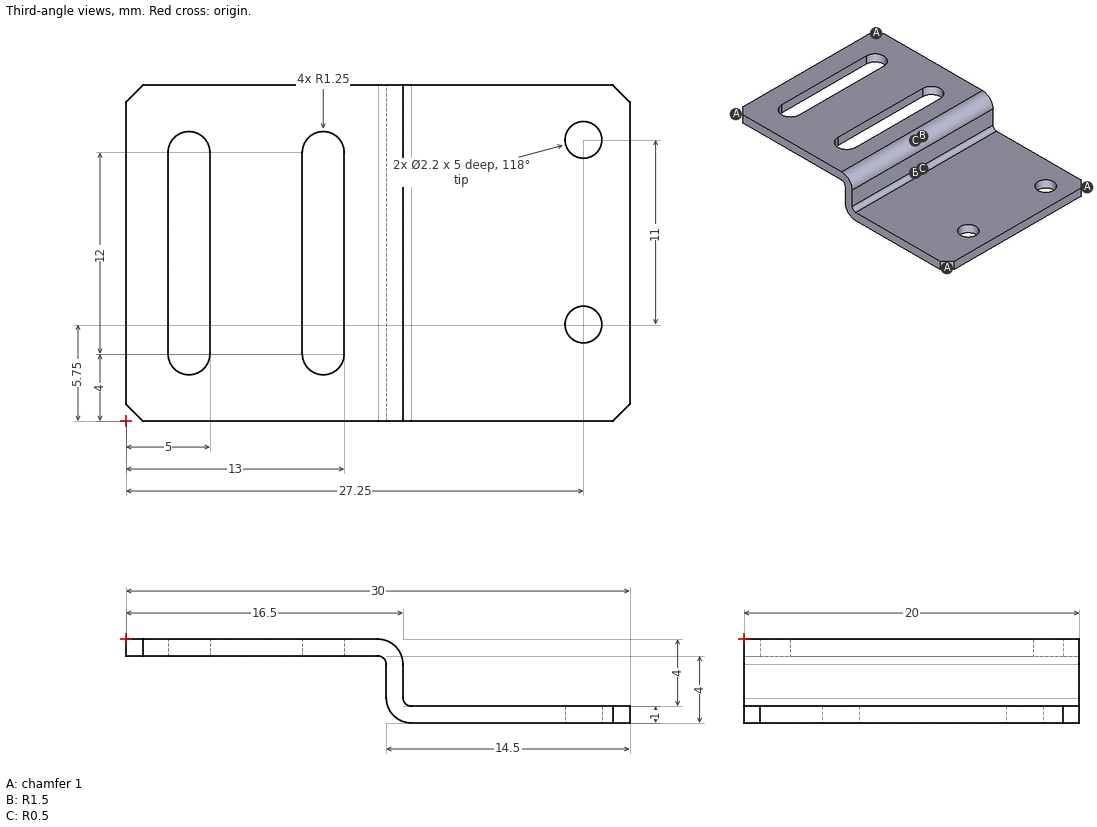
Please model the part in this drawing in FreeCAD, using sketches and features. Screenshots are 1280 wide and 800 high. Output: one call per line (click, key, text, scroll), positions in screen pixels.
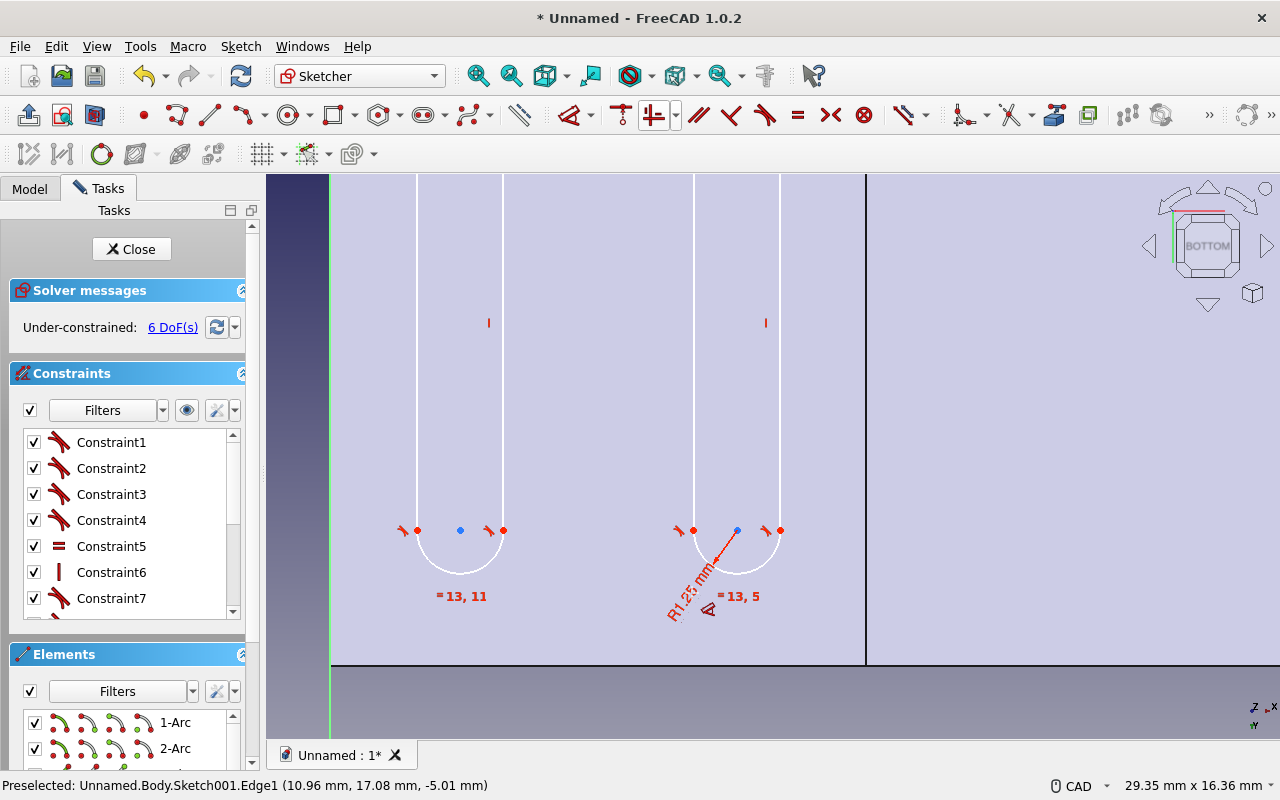
click(694, 406)
click(728, 366)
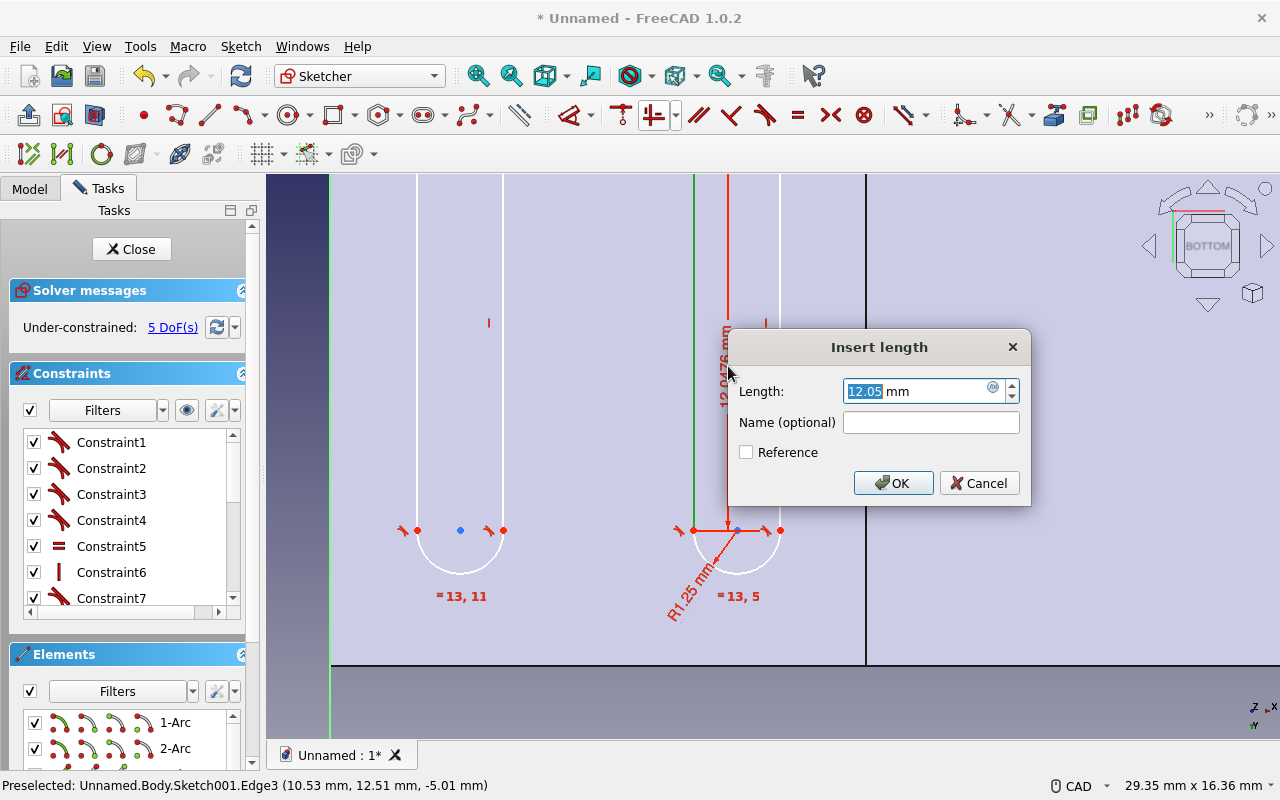
text(12)
key(Return)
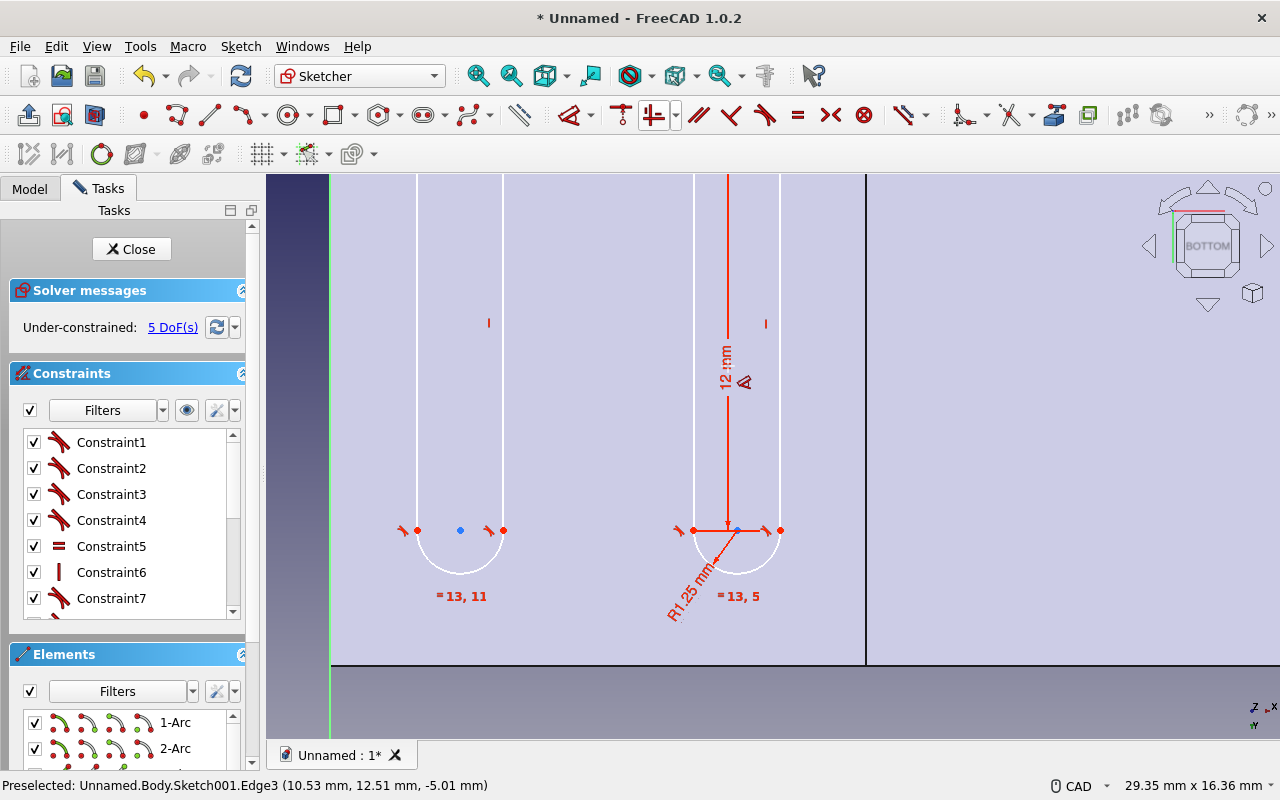
click(417, 406)
click(383, 366)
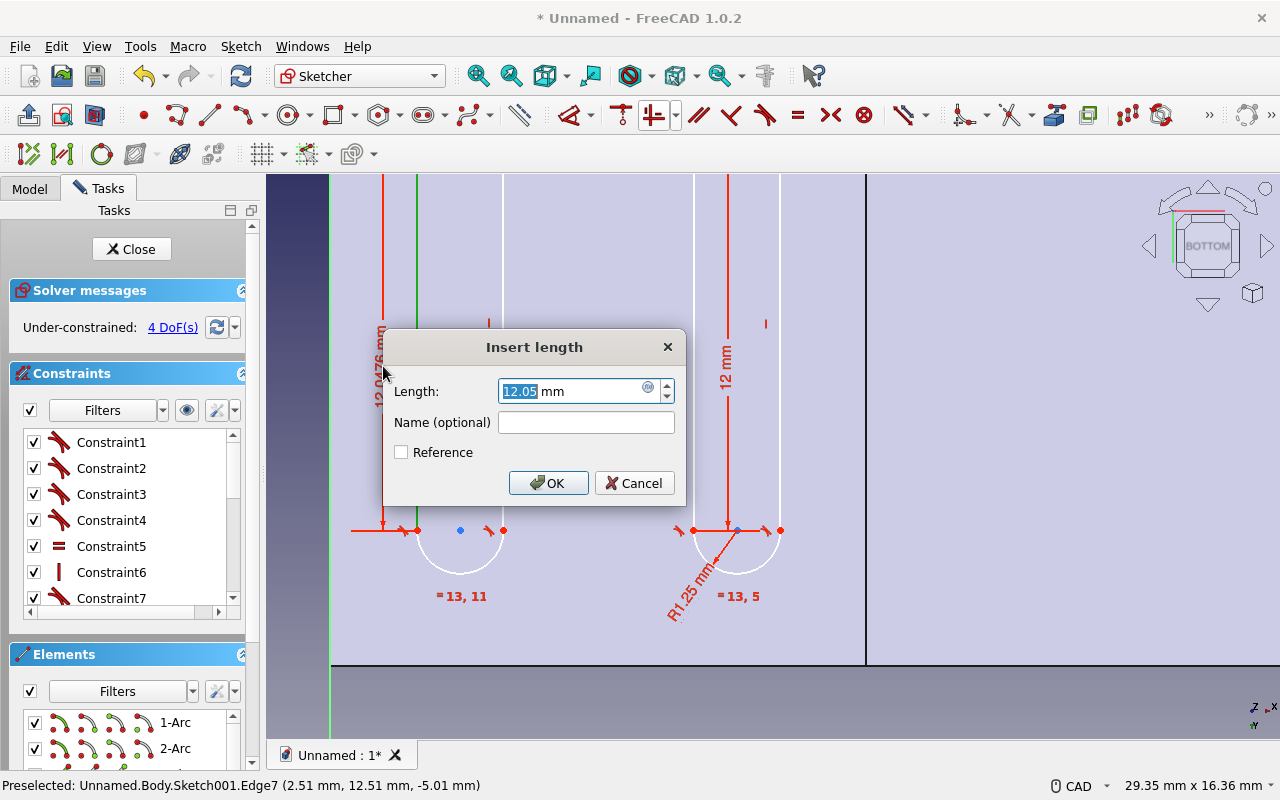
text(12)
key(Return)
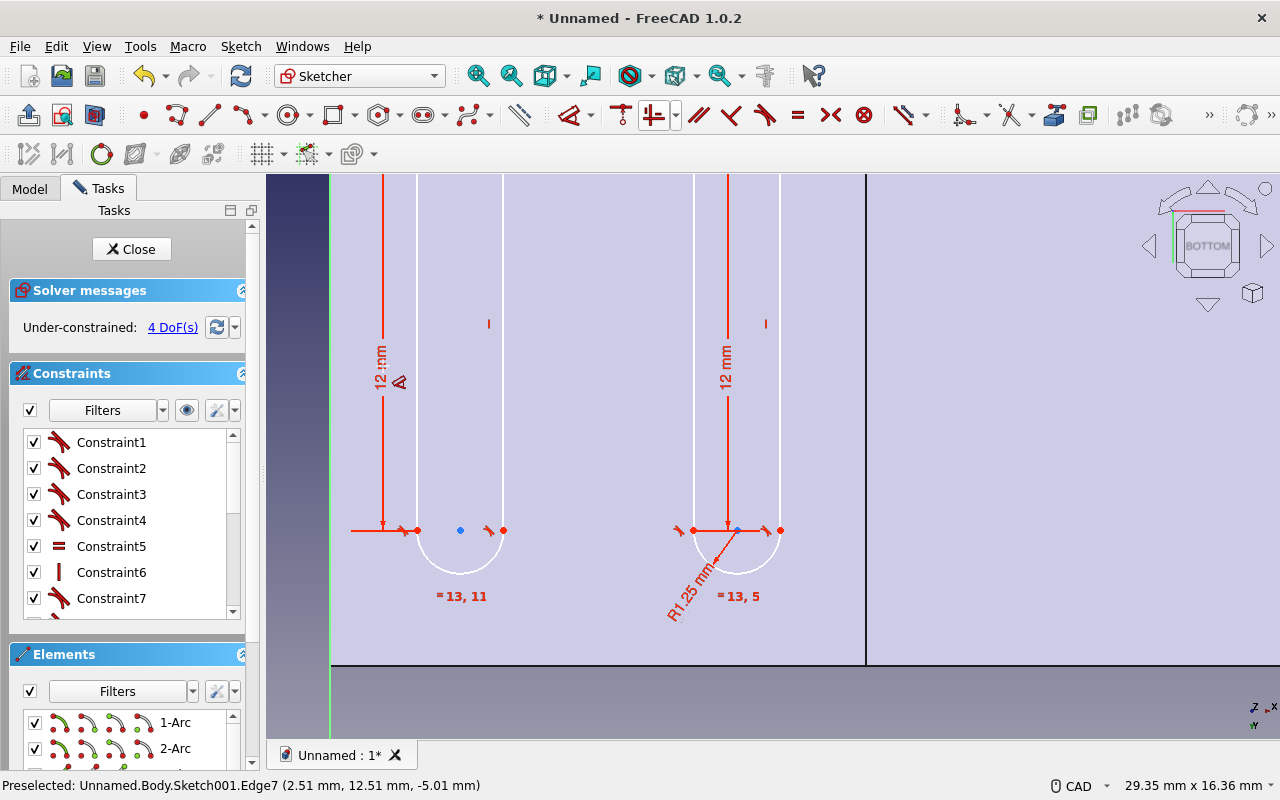
scroll(887, 680, down, 3)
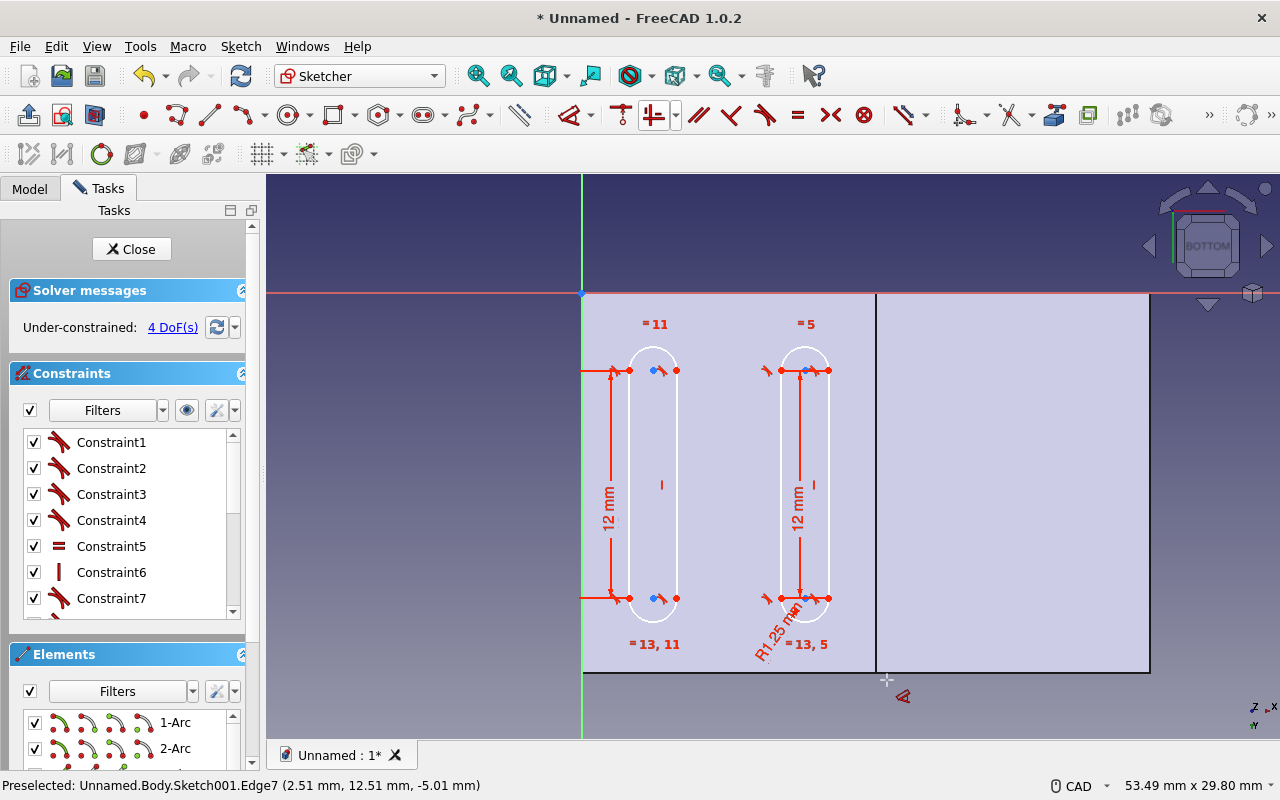
click(829, 371)
click(863, 332)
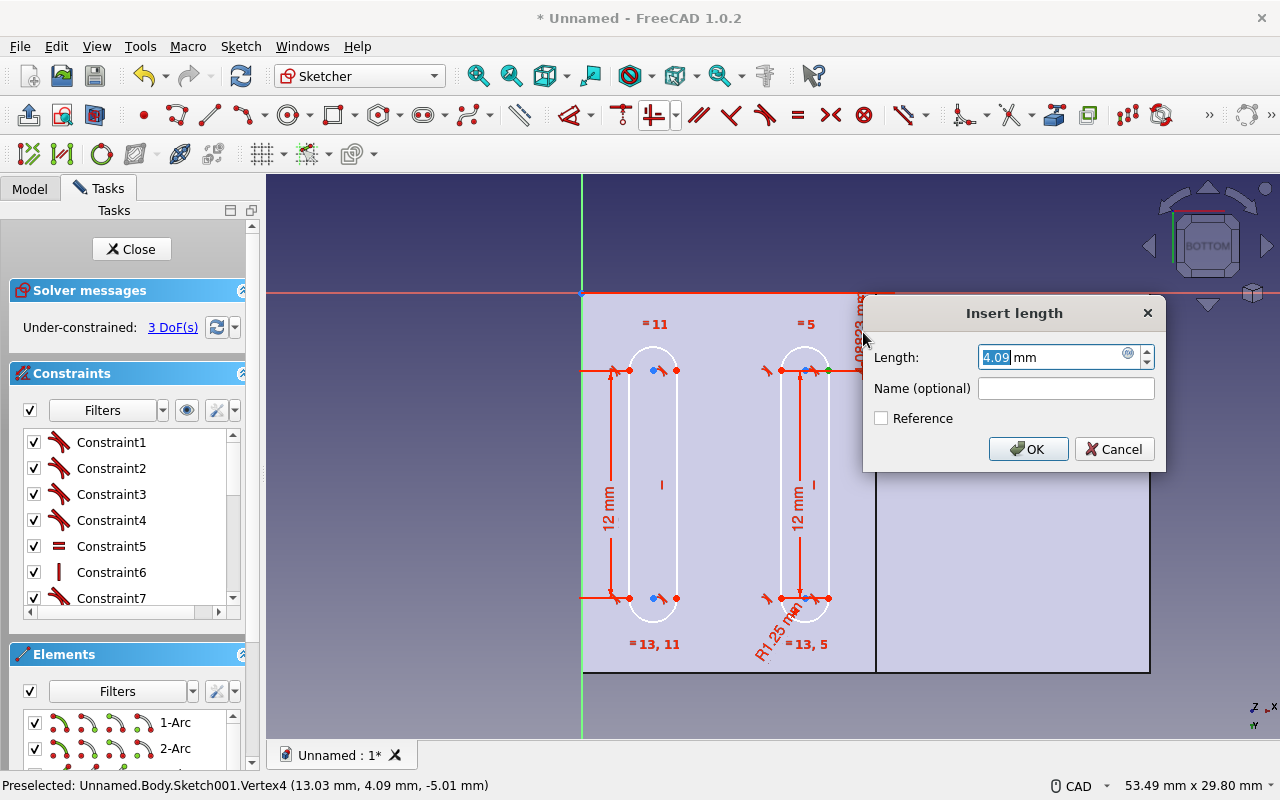
text(4)
key(Return)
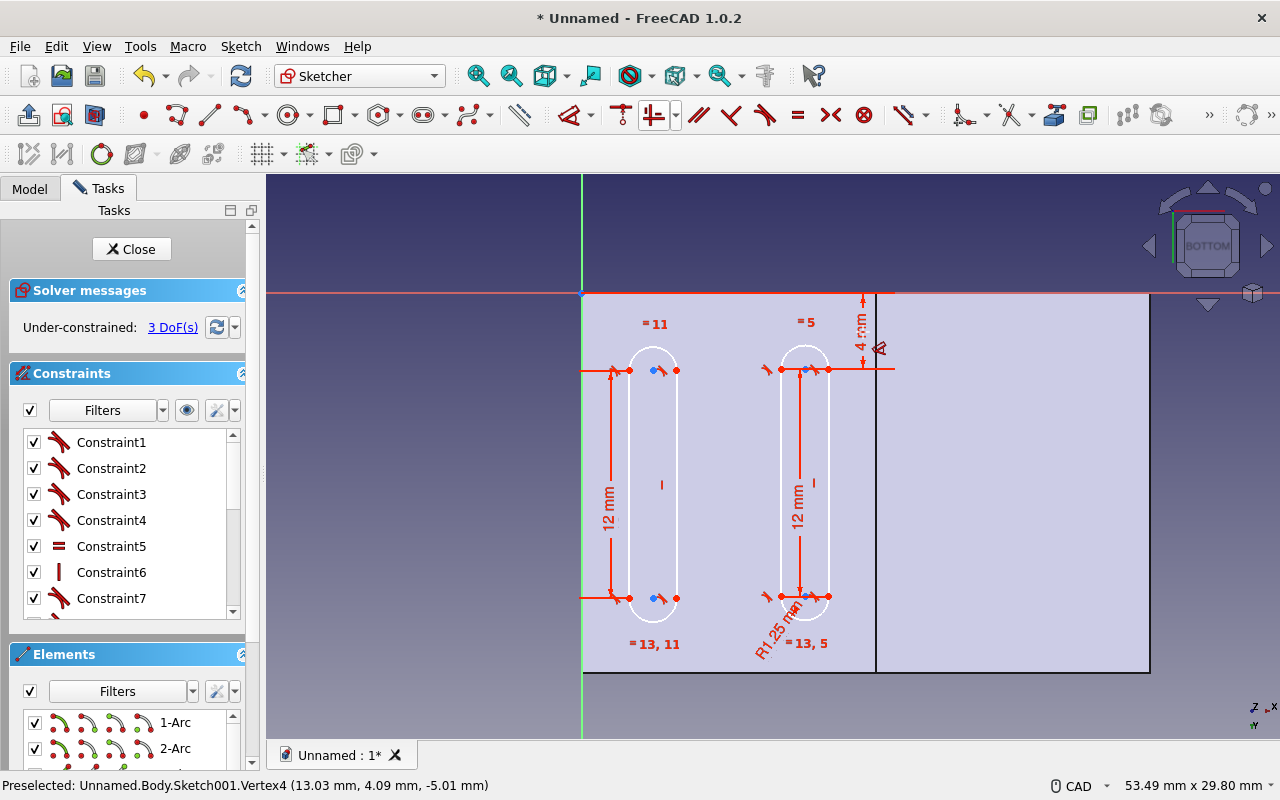
click(677, 598)
click(629, 259)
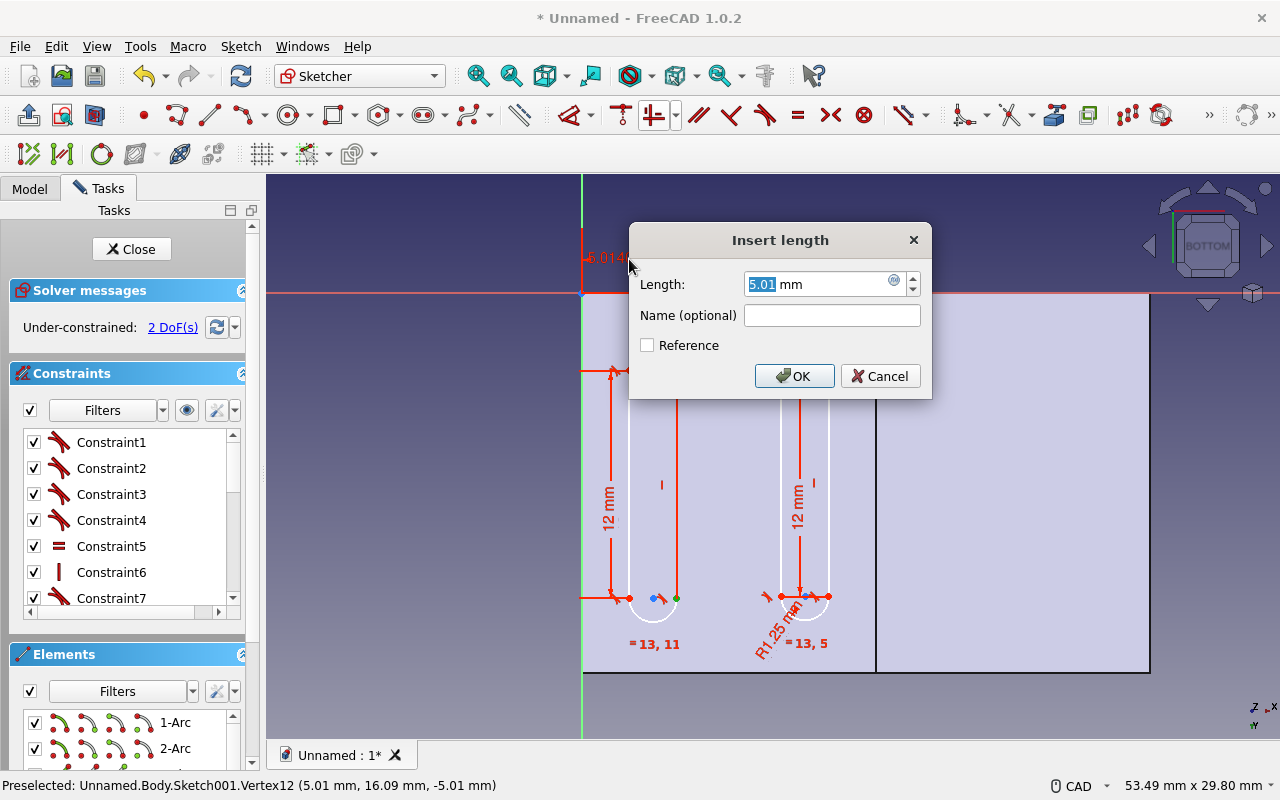
text(5)
key(Return)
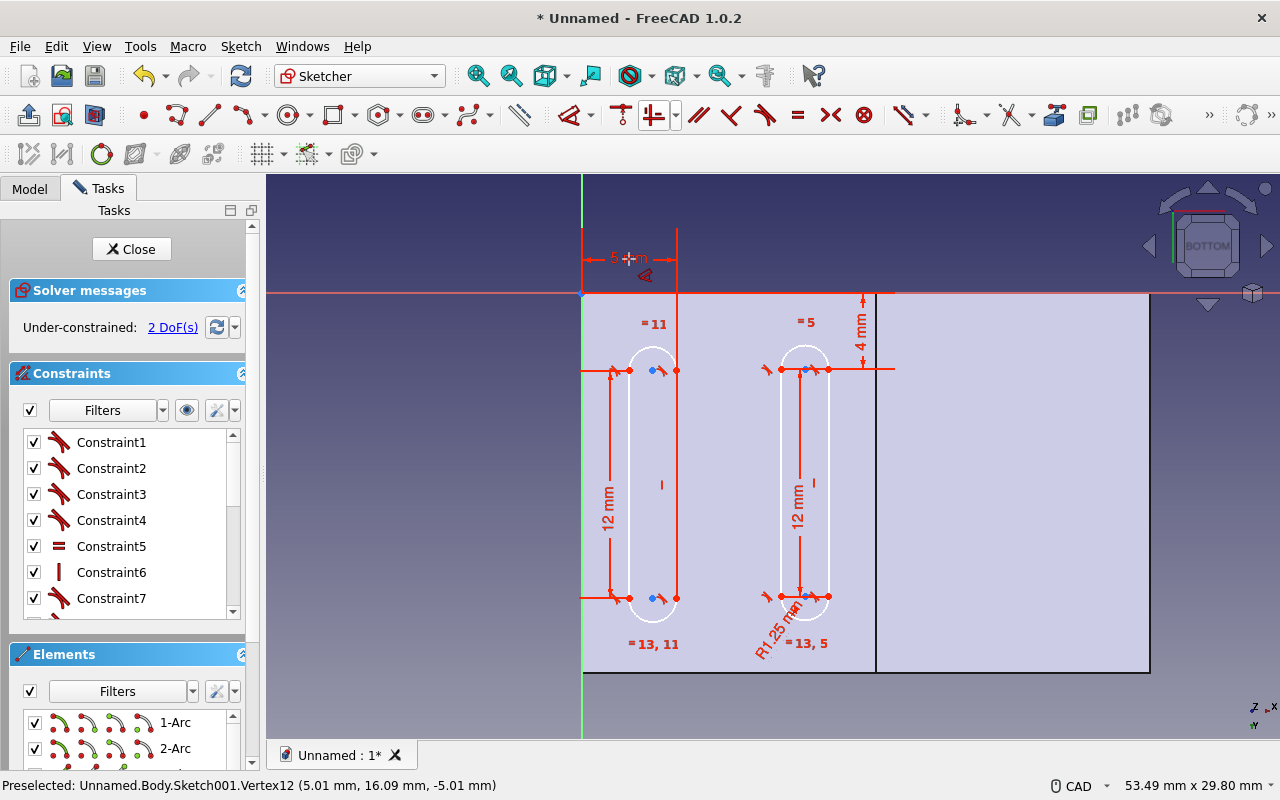
click(677, 371)
click(548, 332)